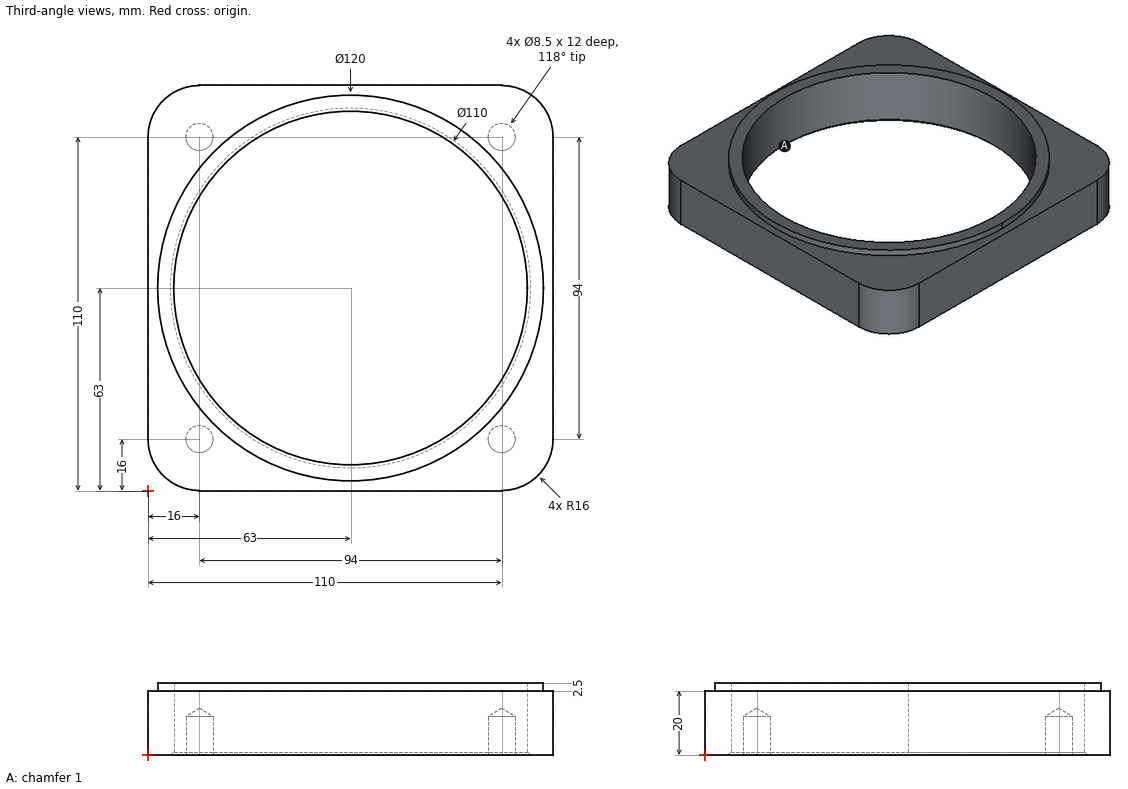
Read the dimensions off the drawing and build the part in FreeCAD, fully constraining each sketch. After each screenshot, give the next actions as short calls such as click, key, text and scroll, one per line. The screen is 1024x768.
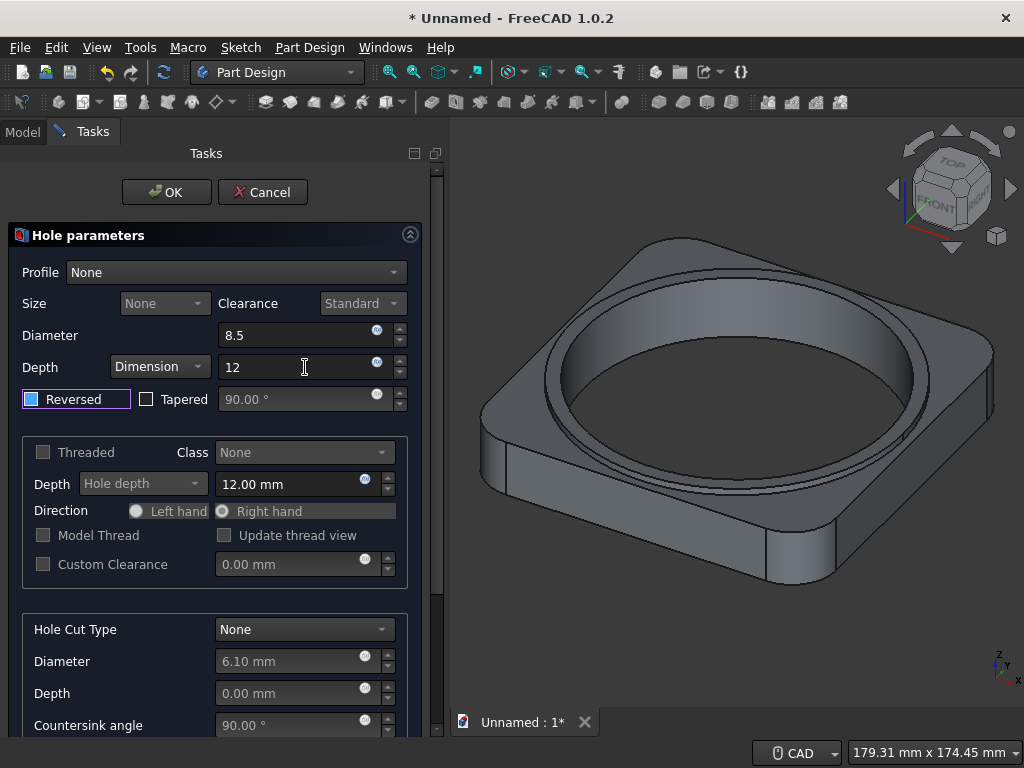
click(30, 399)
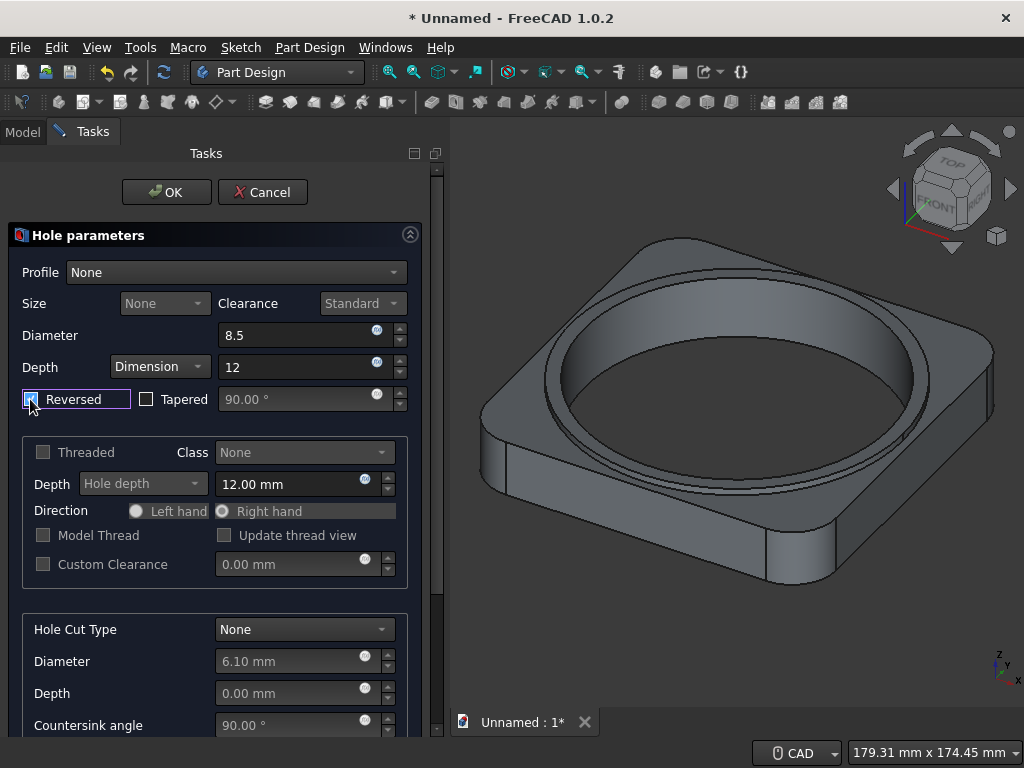
click(167, 192)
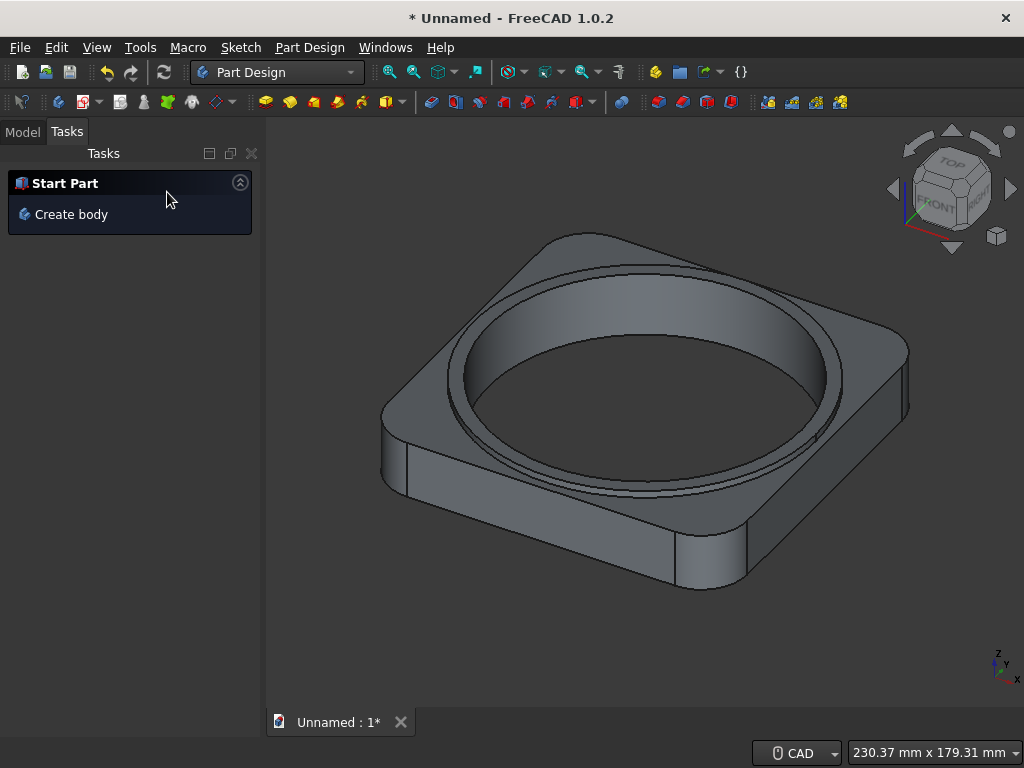
key(0)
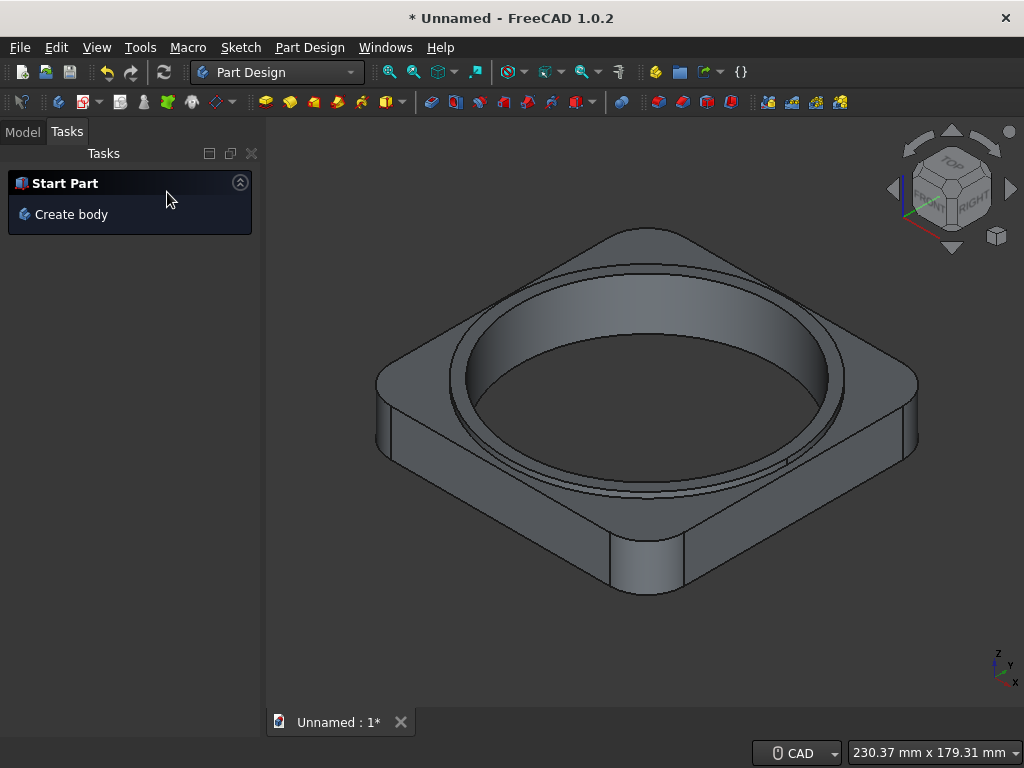
key(2)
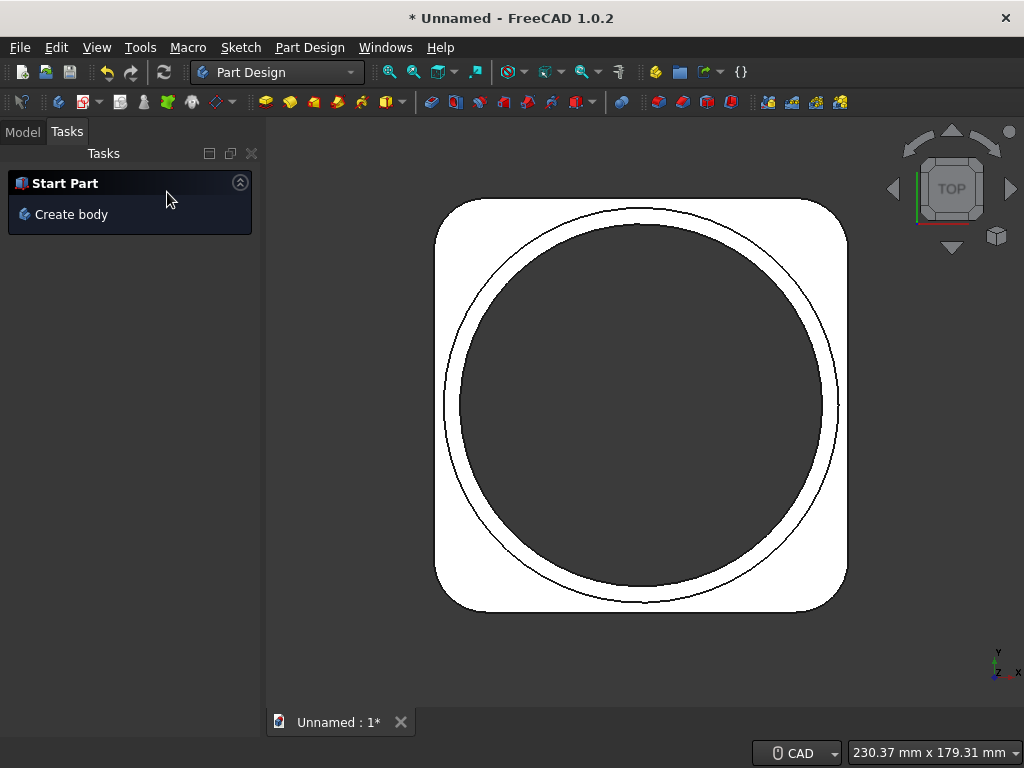
key(1)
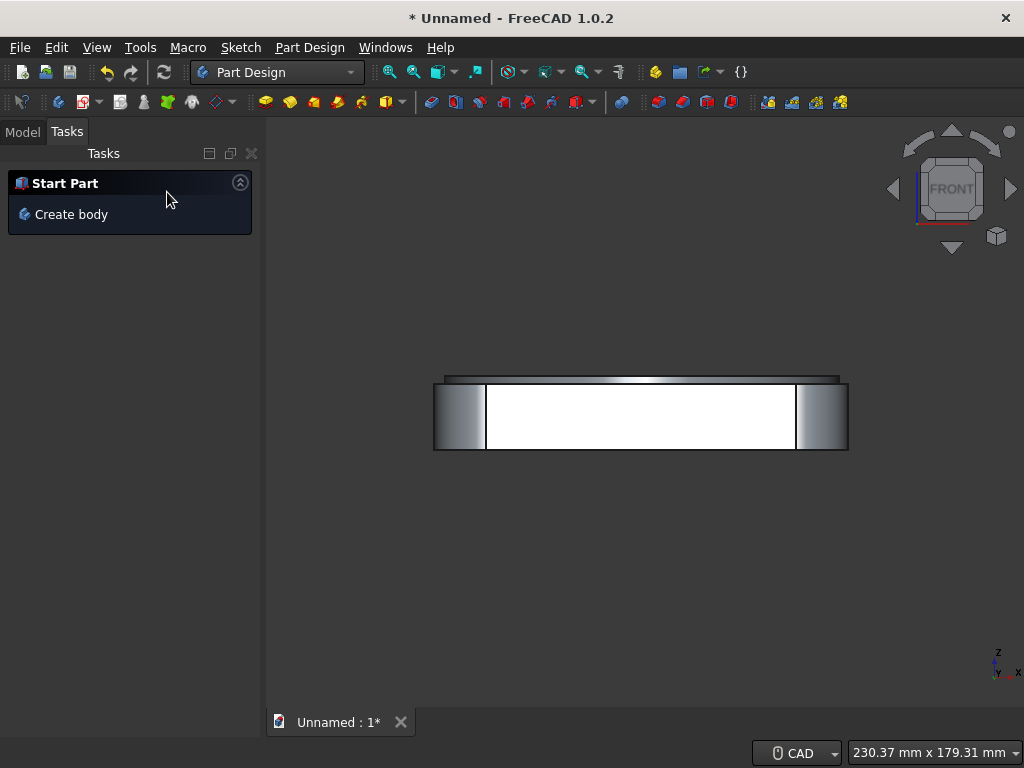
key(3)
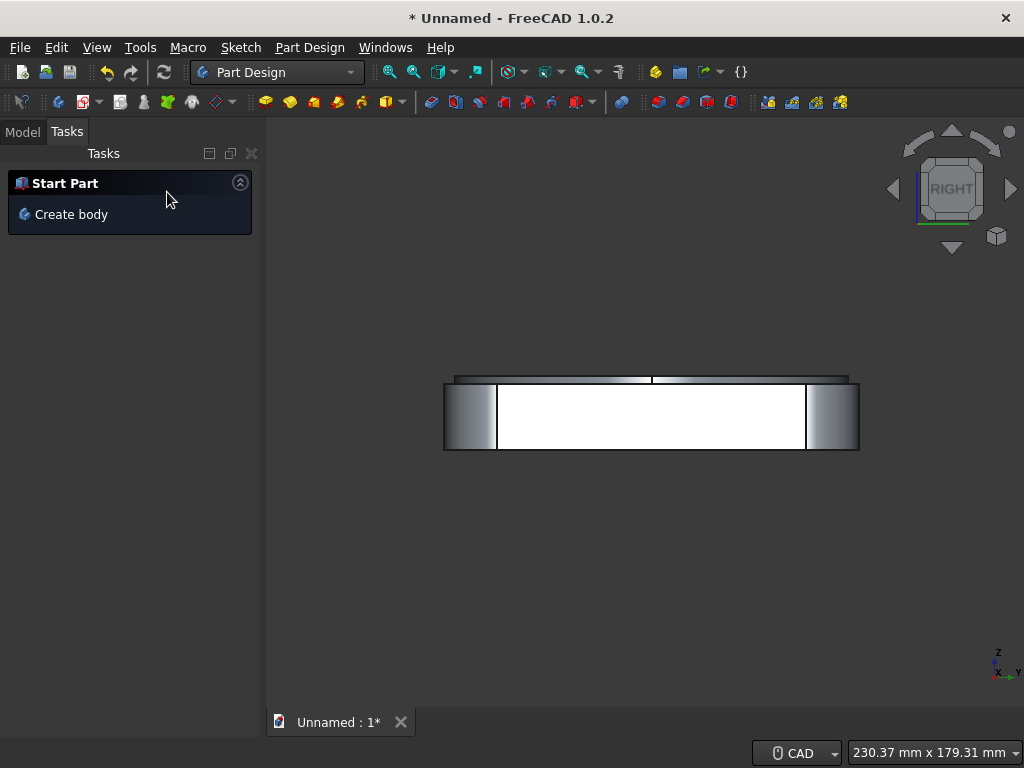
key(5)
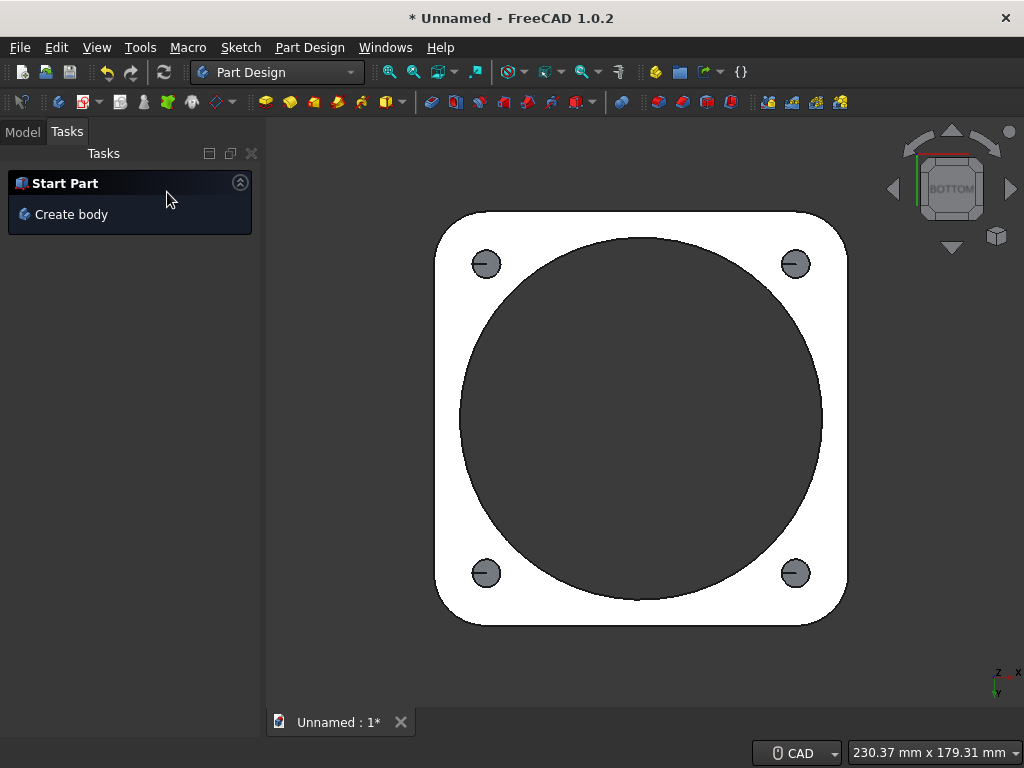
click(495, 524)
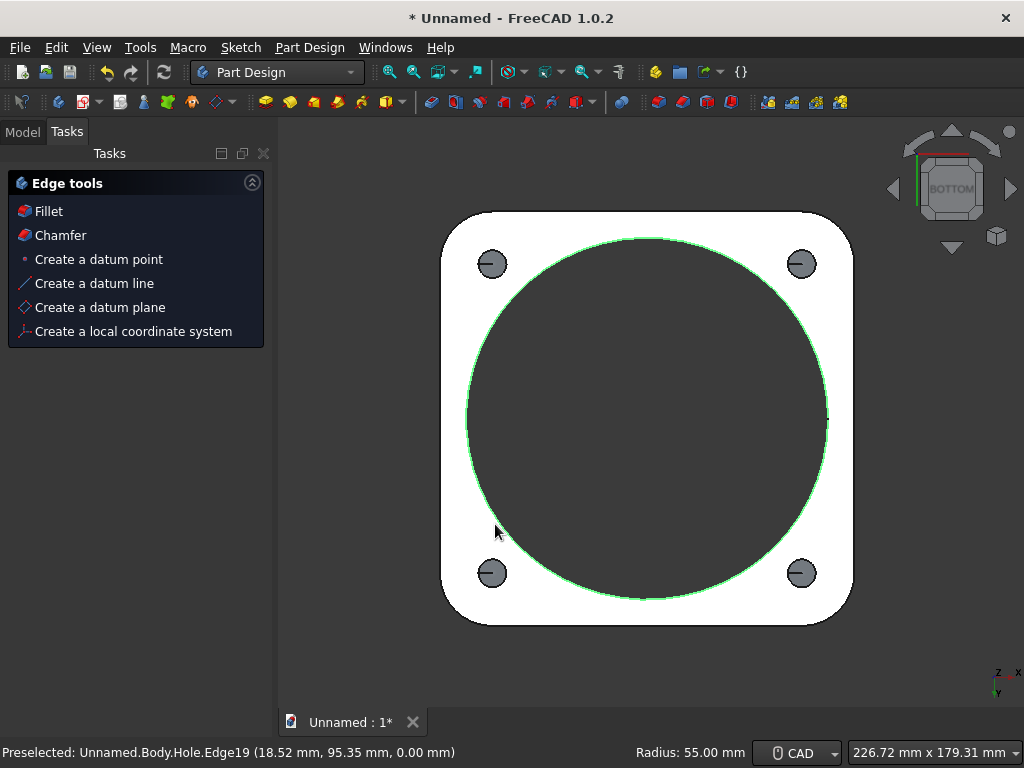
click(684, 102)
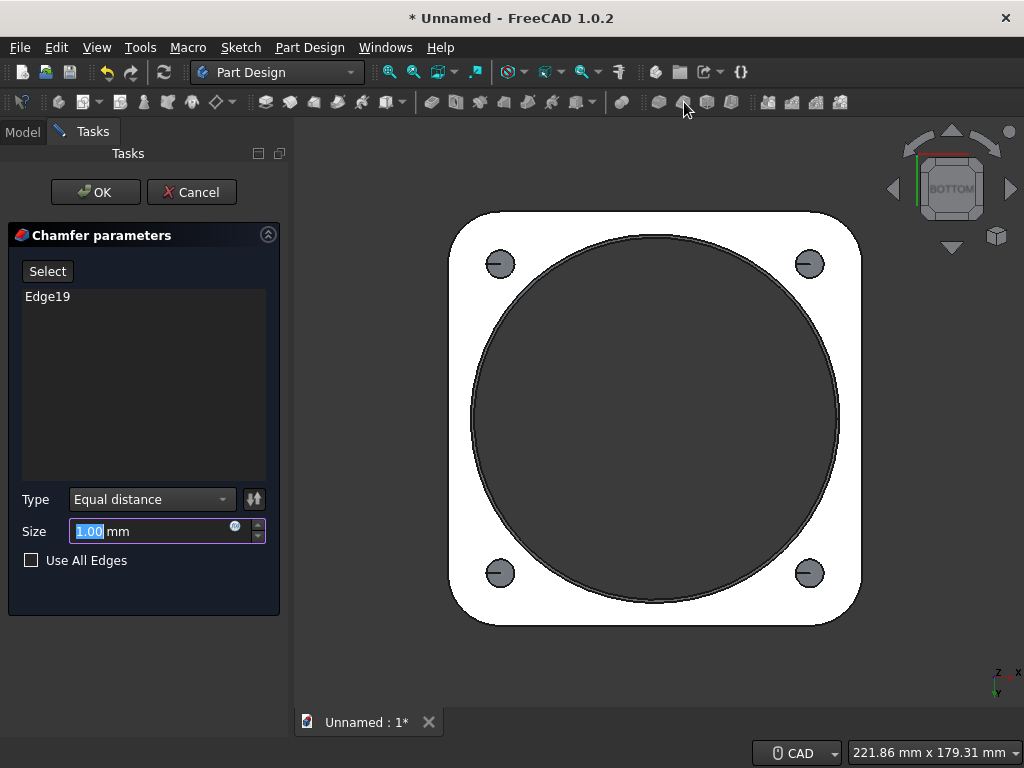
text(1)
key(Tab)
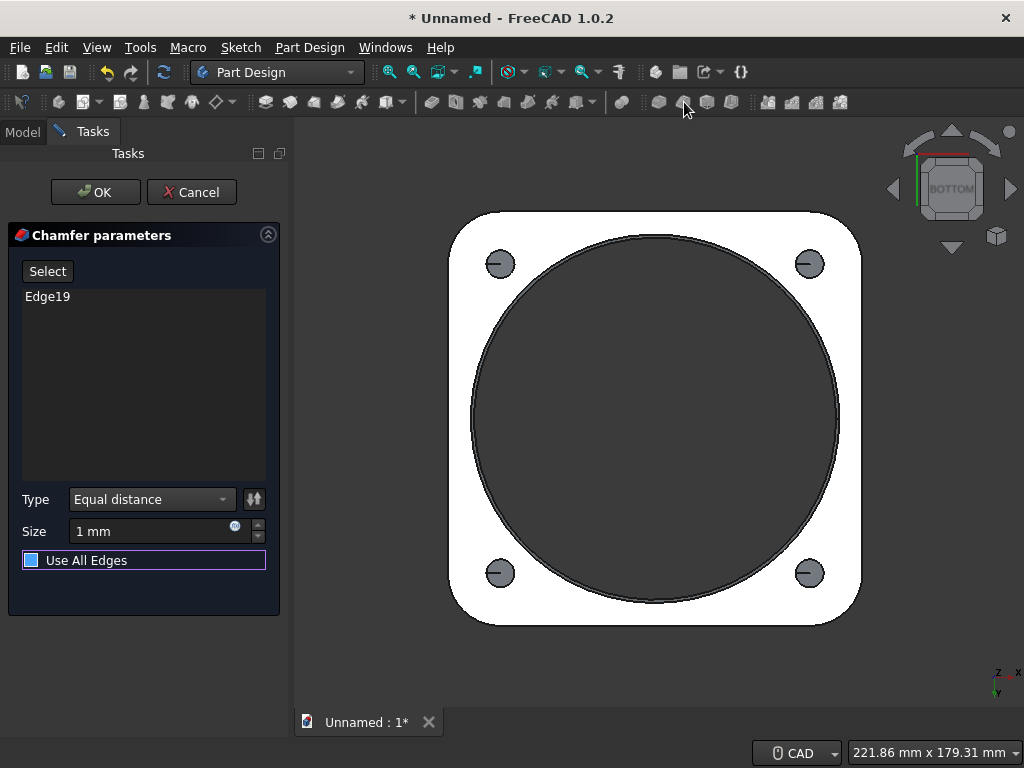
click(96, 192)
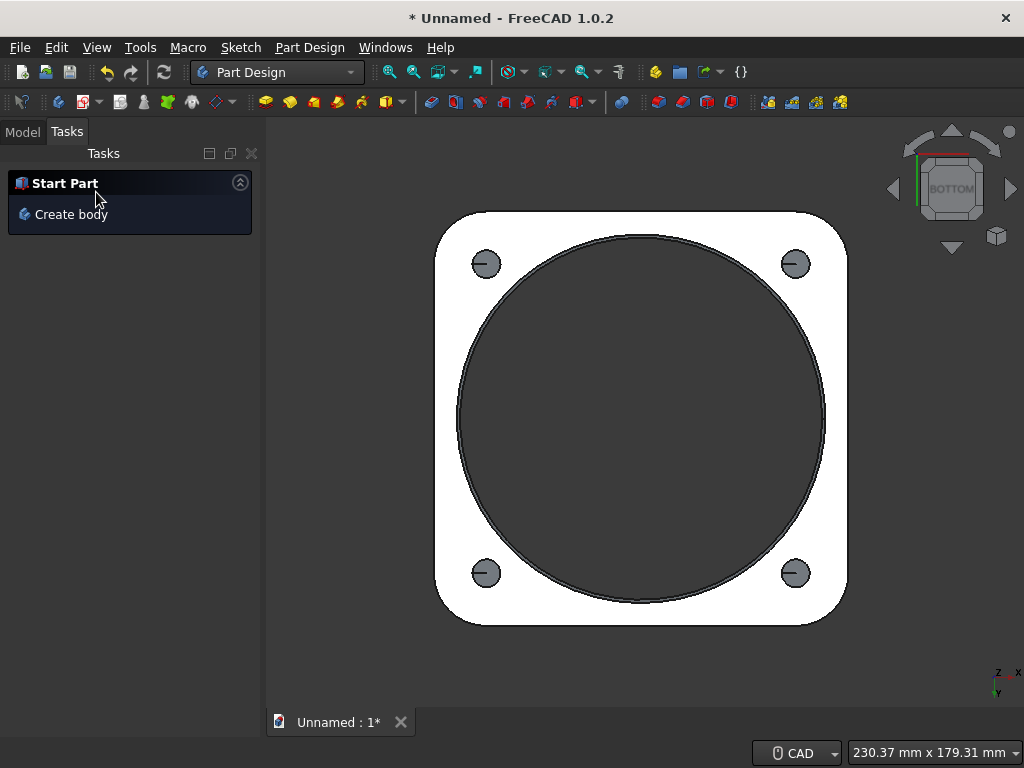
key(0)